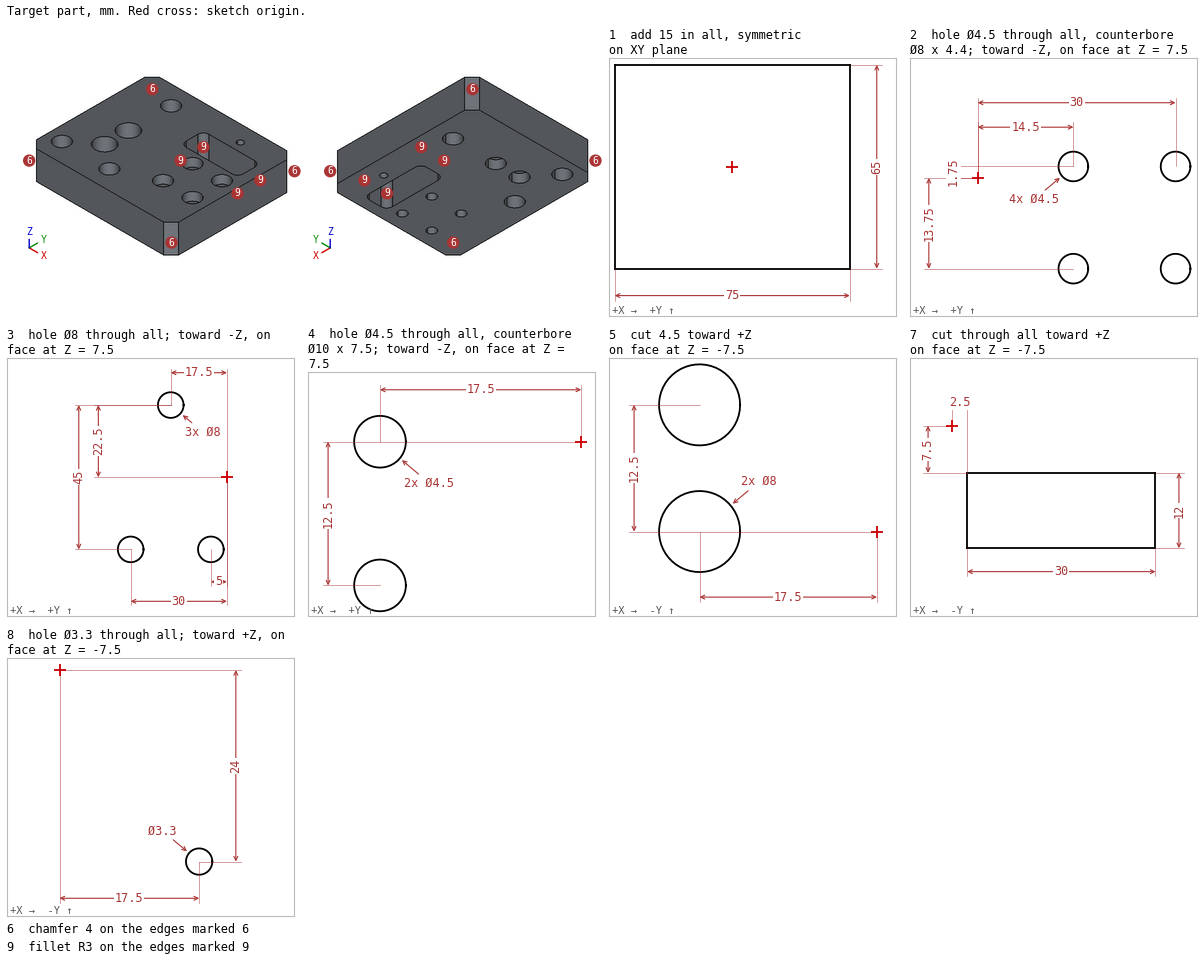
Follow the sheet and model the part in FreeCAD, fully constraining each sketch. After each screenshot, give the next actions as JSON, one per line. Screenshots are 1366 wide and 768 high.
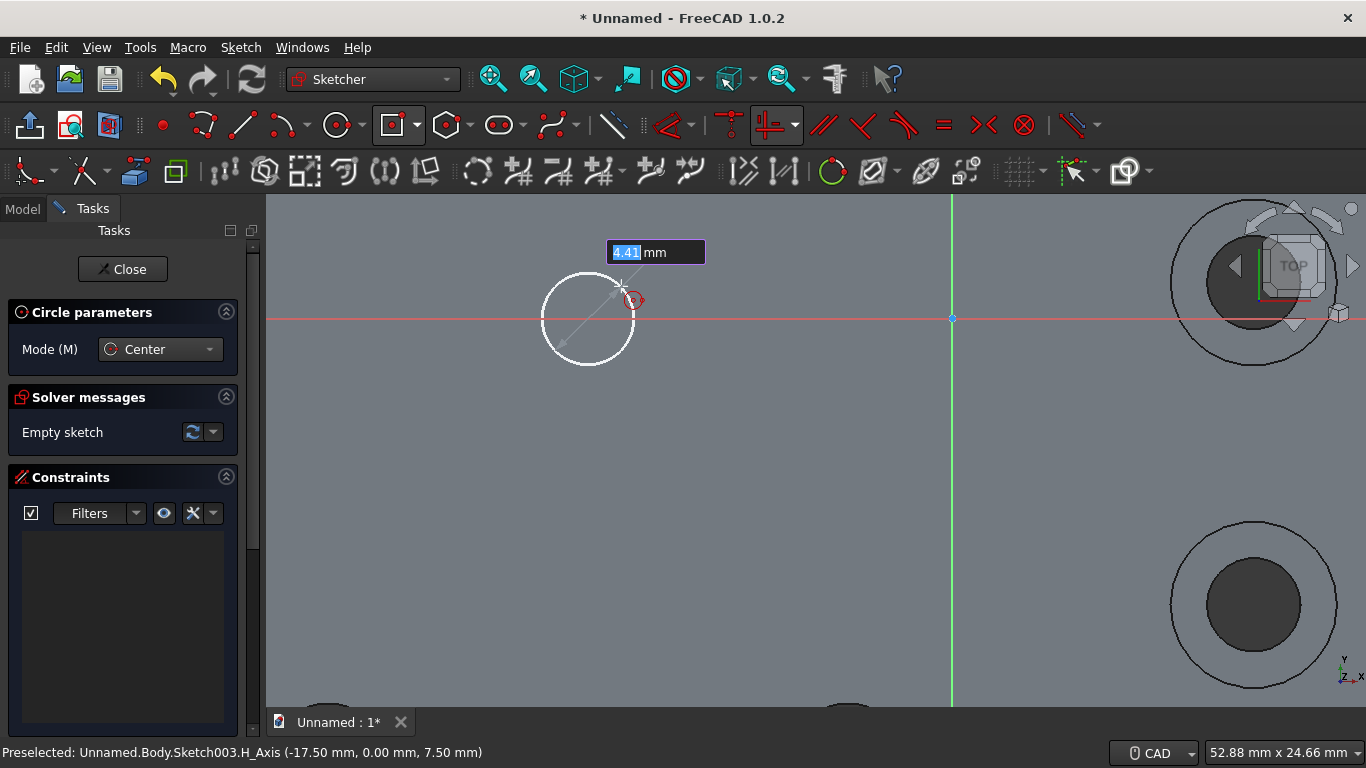
{"action": "type", "text": "4.5"}
{"action": "key", "text": "Return"}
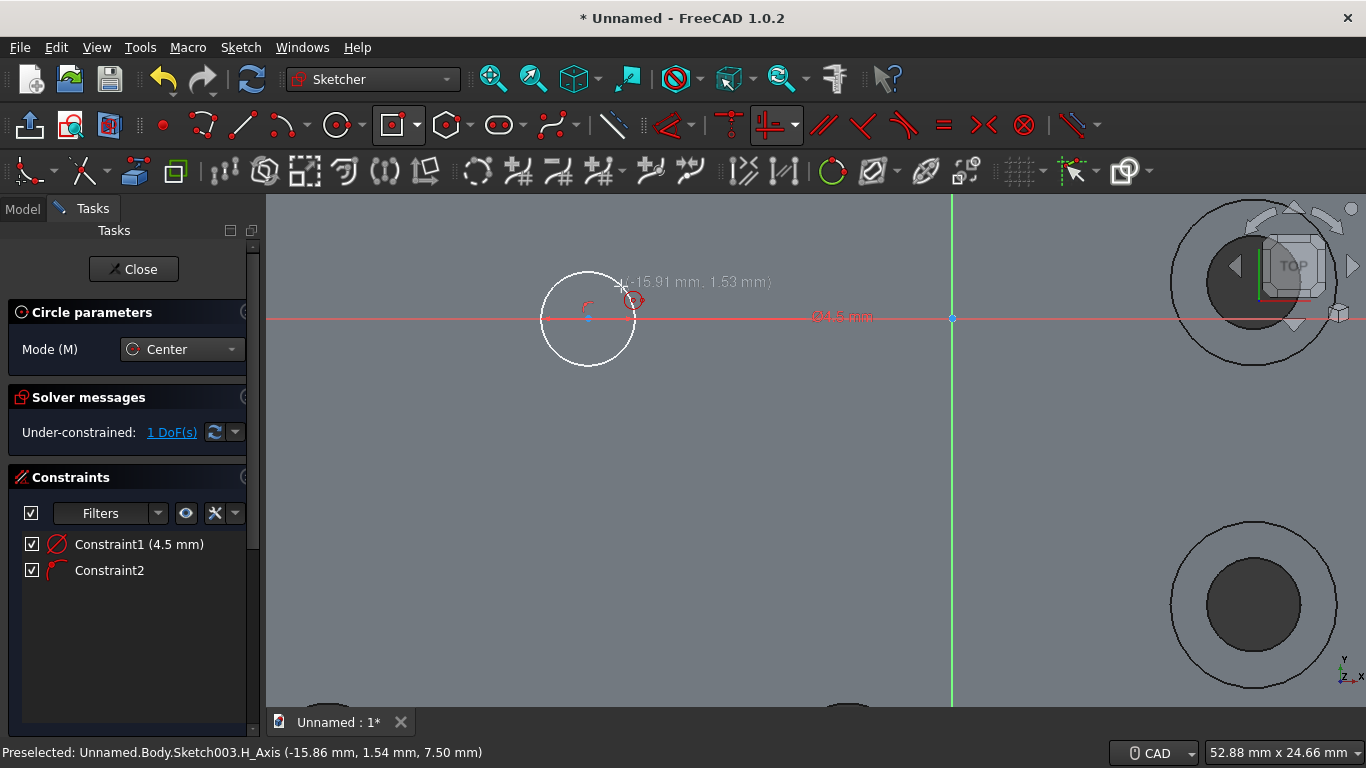
{"action": "left_click", "coordinate": [588, 579]}
{"action": "mouse_move", "coordinate": [621, 546]}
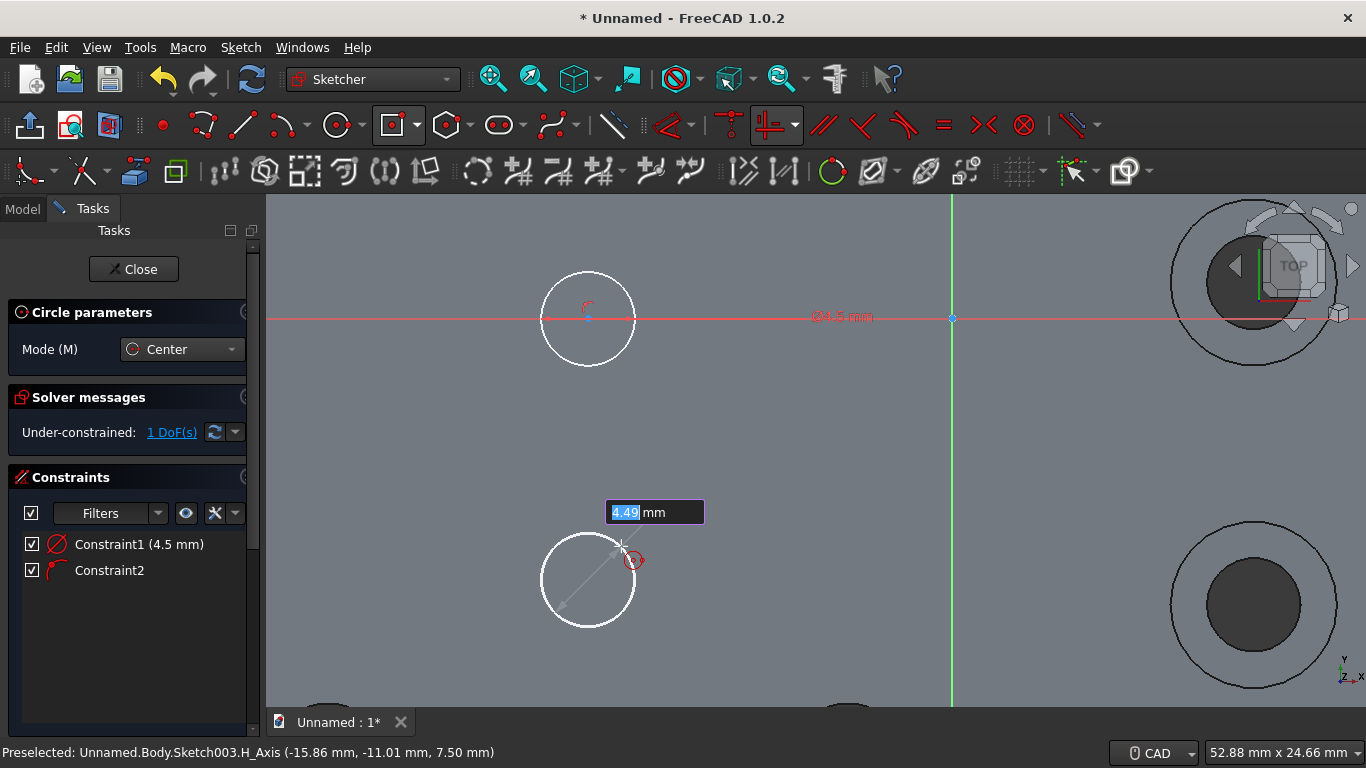
{"action": "type", "text": "4.5"}
{"action": "key", "text": "Return"}
{"action": "key", "text": "Escape"}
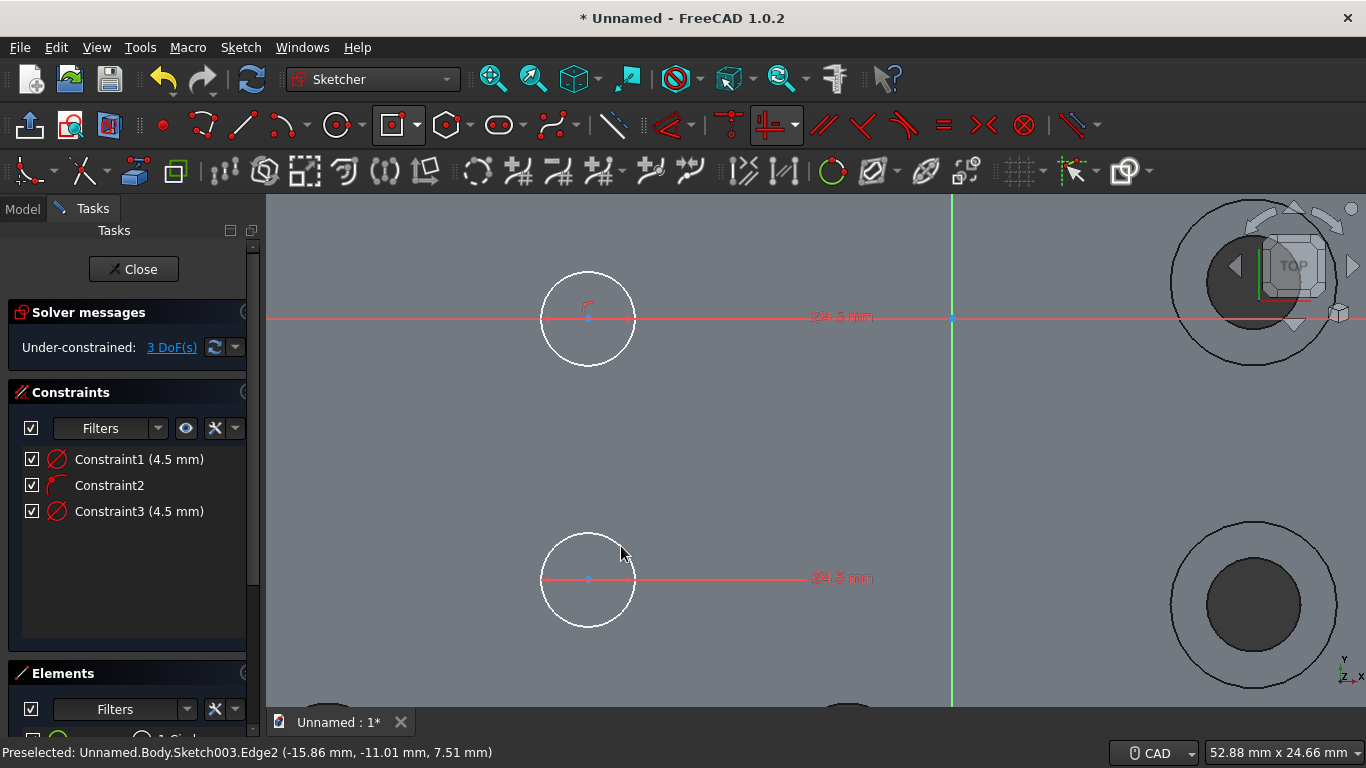
{"action": "left_click", "coordinate": [588, 319]}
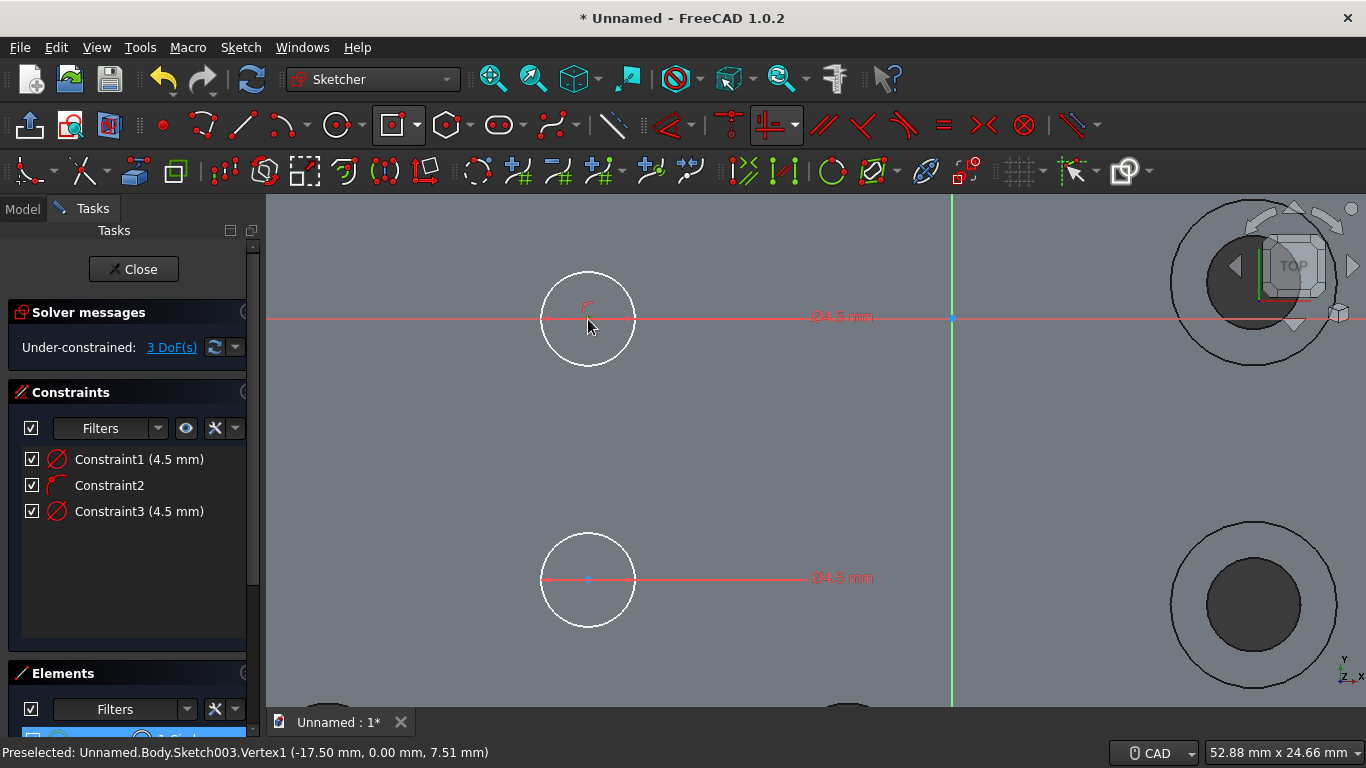
{"action": "left_click", "coordinate": [588, 580]}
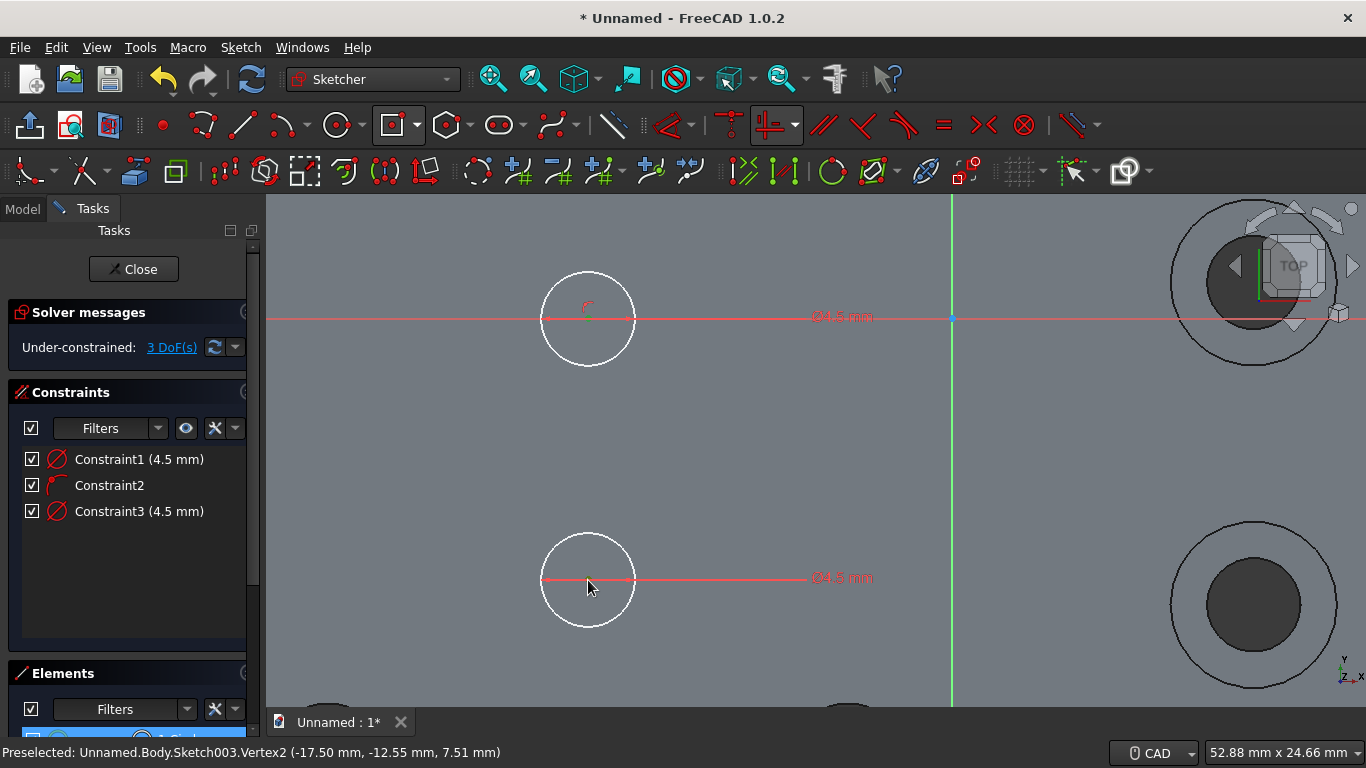
{"action": "left_click", "coordinate": [798, 126]}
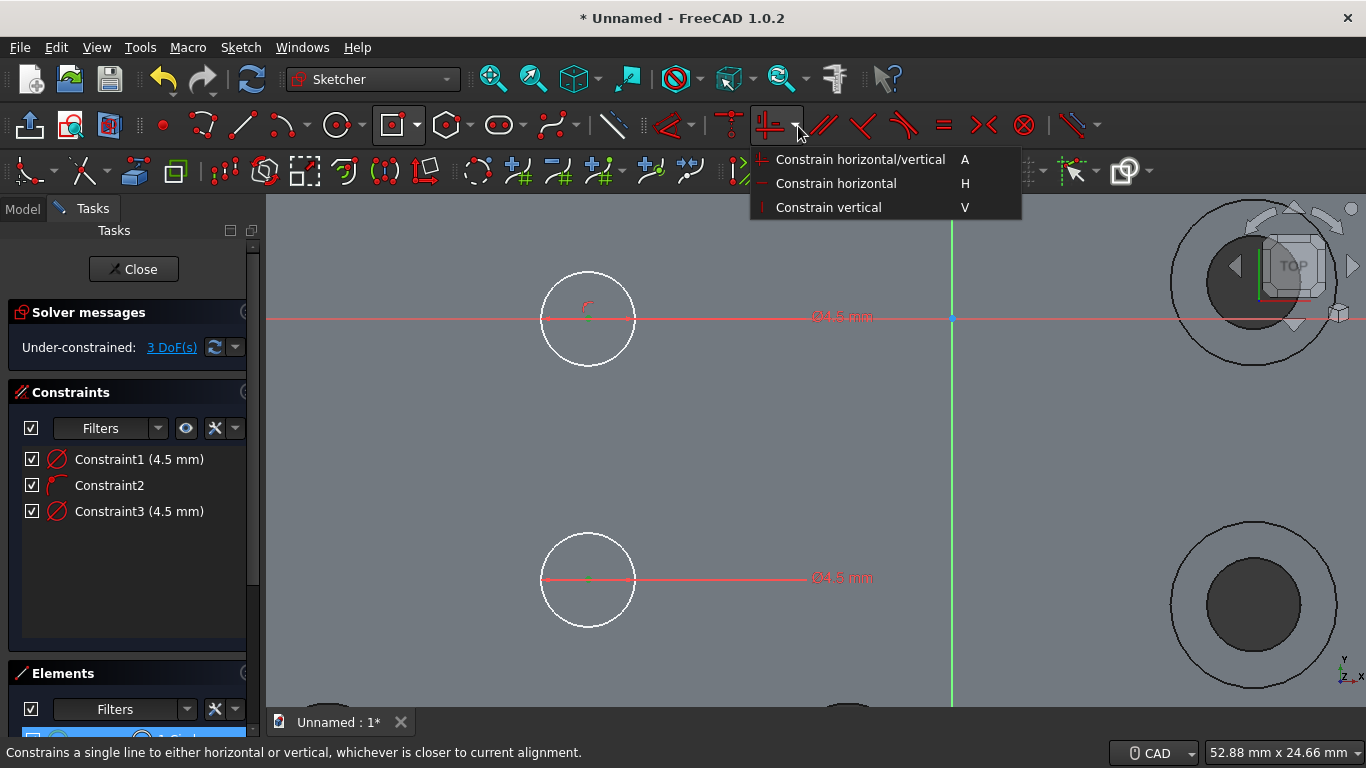
{"action": "left_click", "coordinate": [886, 207]}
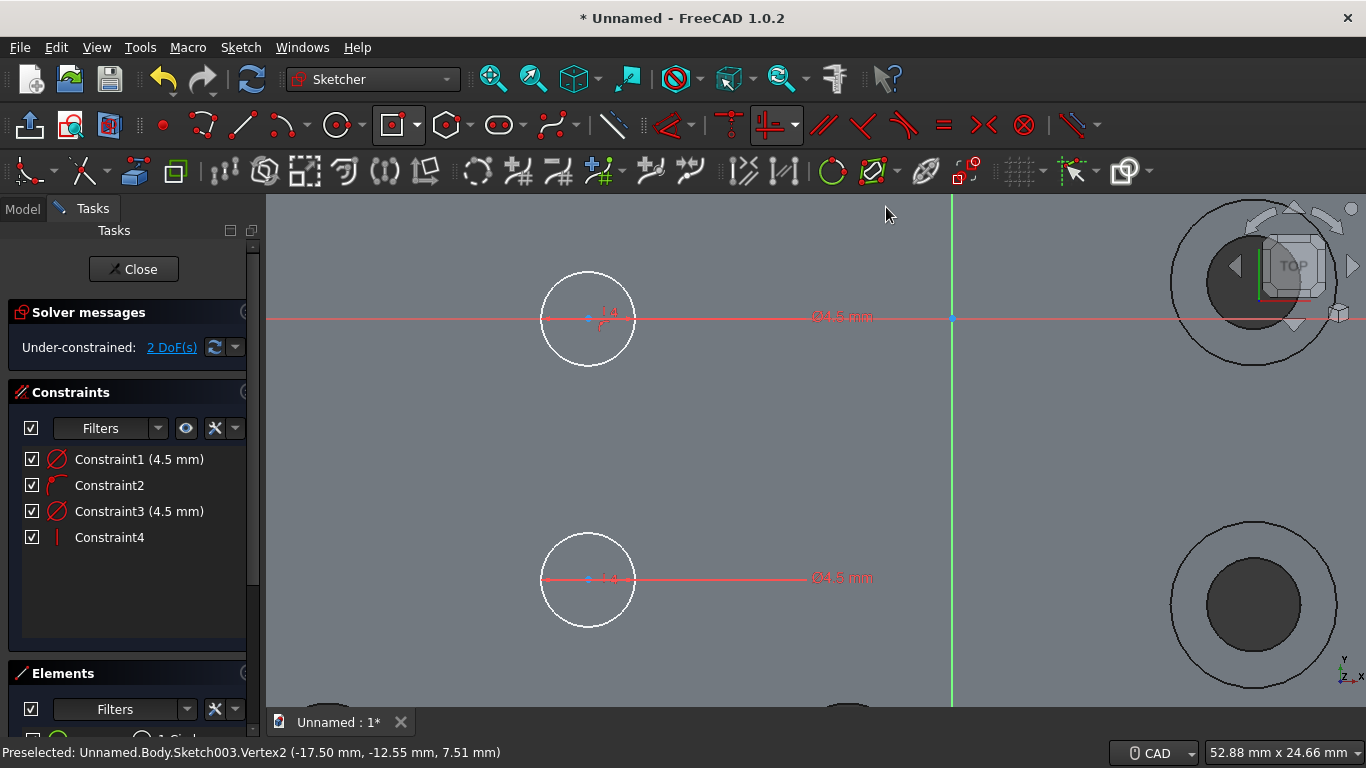
{"action": "left_click", "coordinate": [588, 319]}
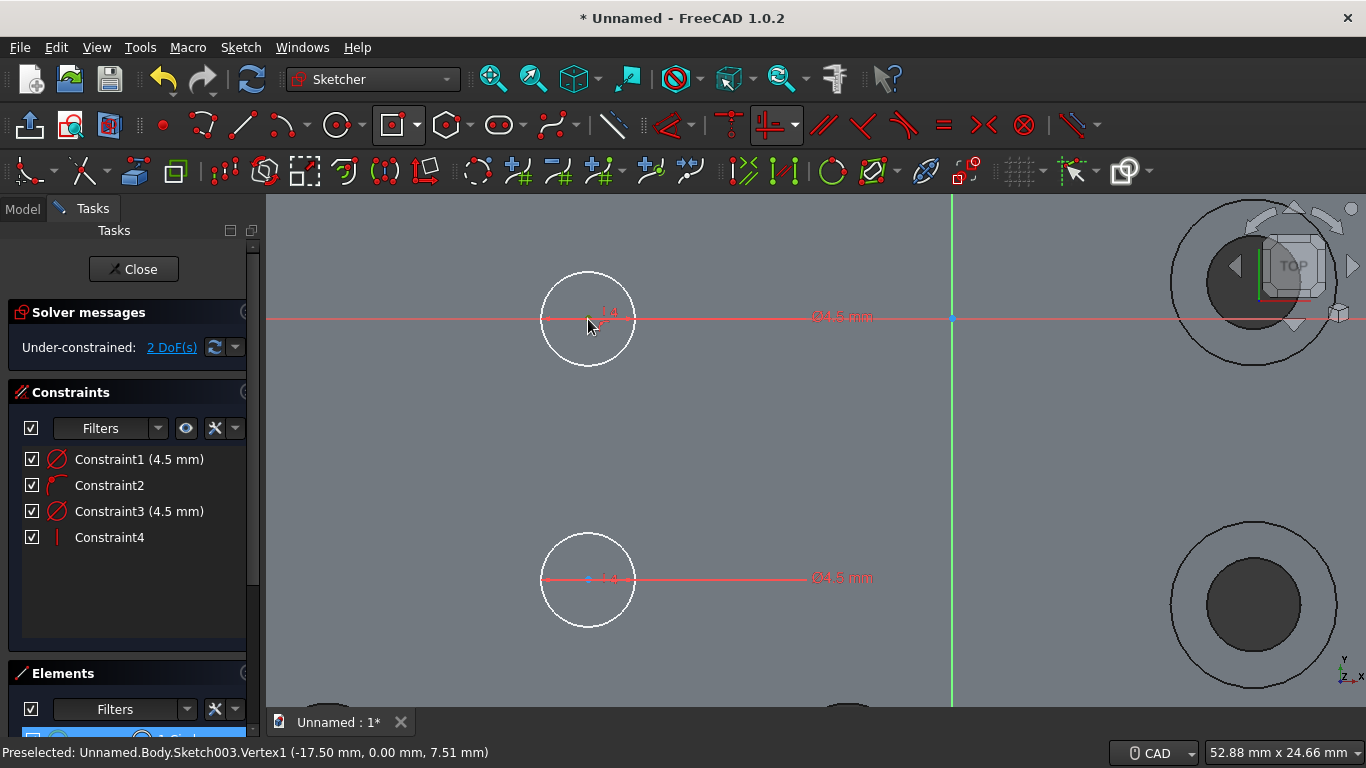
{"action": "key", "text": "l"}